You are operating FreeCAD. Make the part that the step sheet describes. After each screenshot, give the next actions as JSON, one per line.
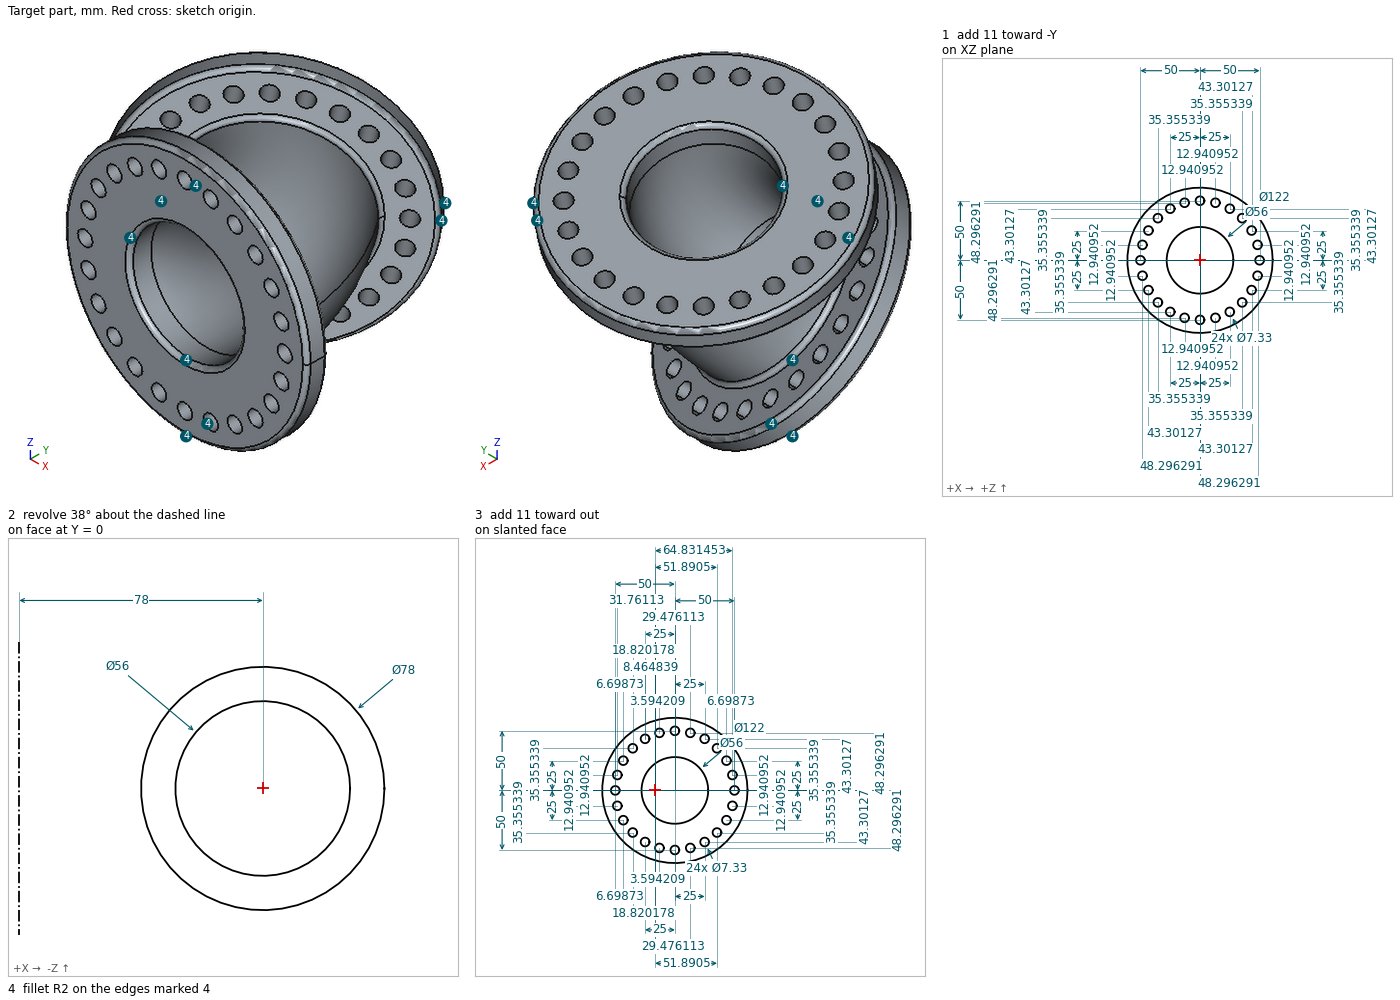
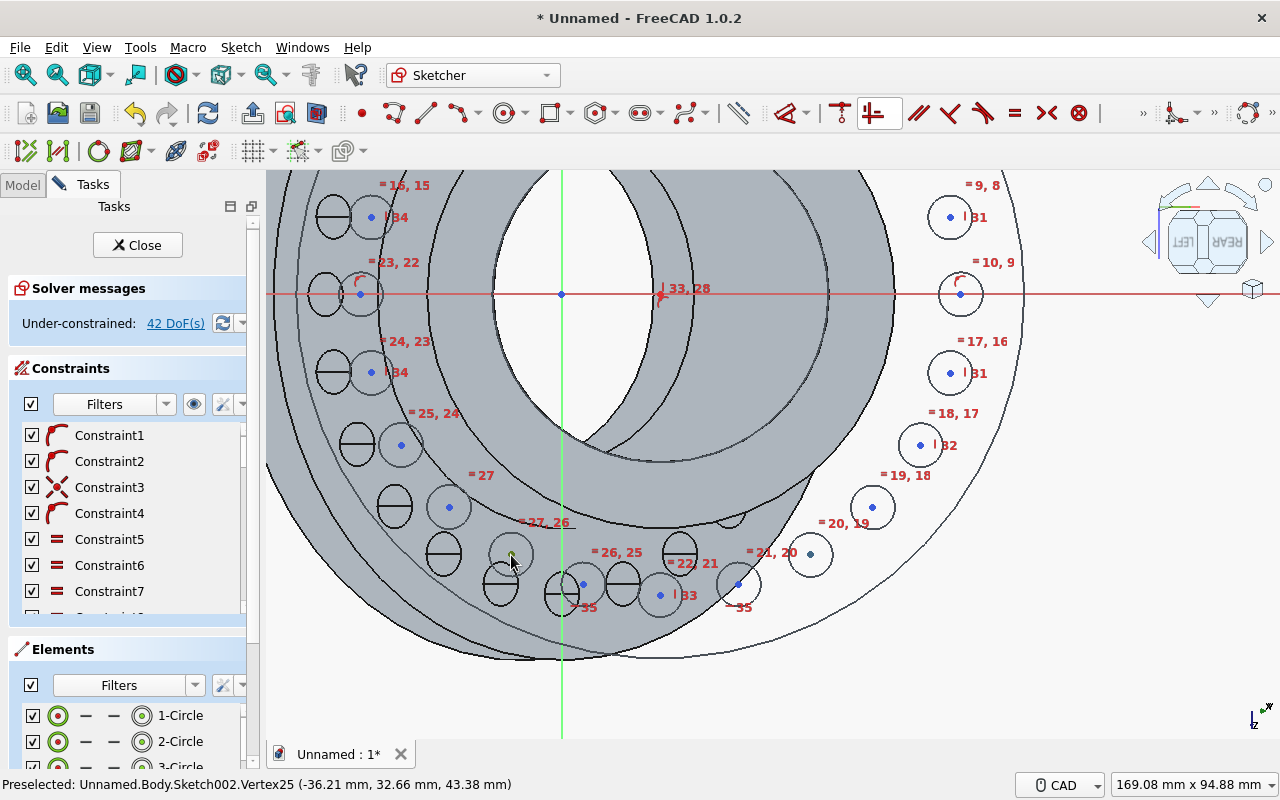
{"action": "left_click", "coordinate": [896, 114]}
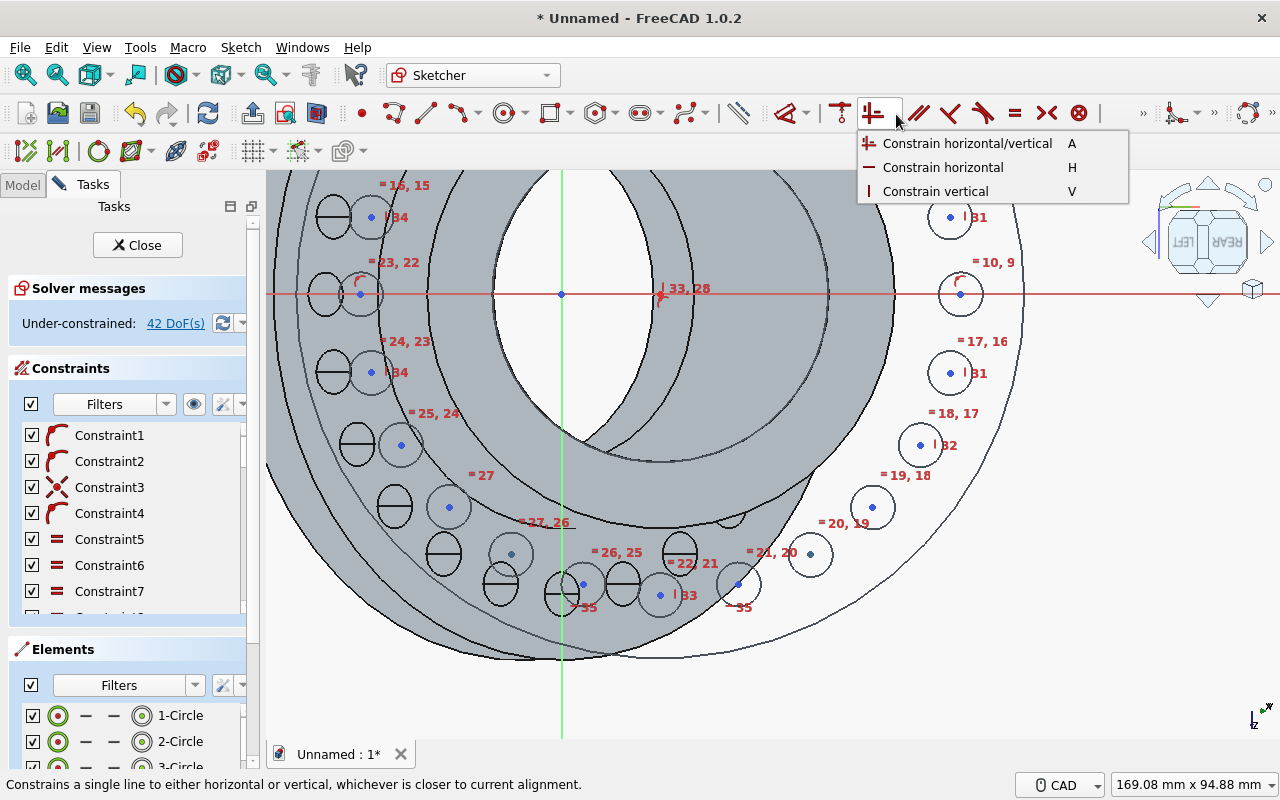
{"action": "left_click", "coordinate": [993, 167]}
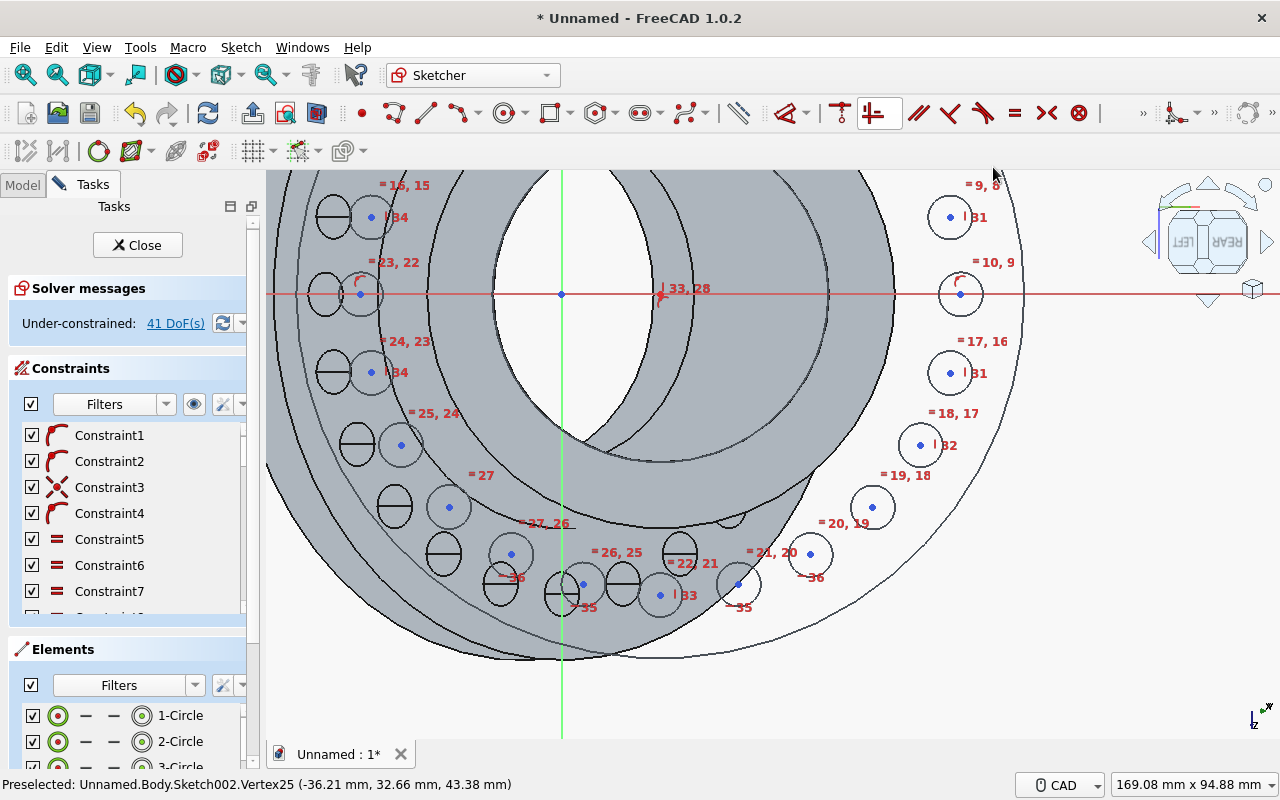
{"action": "left_click", "coordinate": [786, 114]}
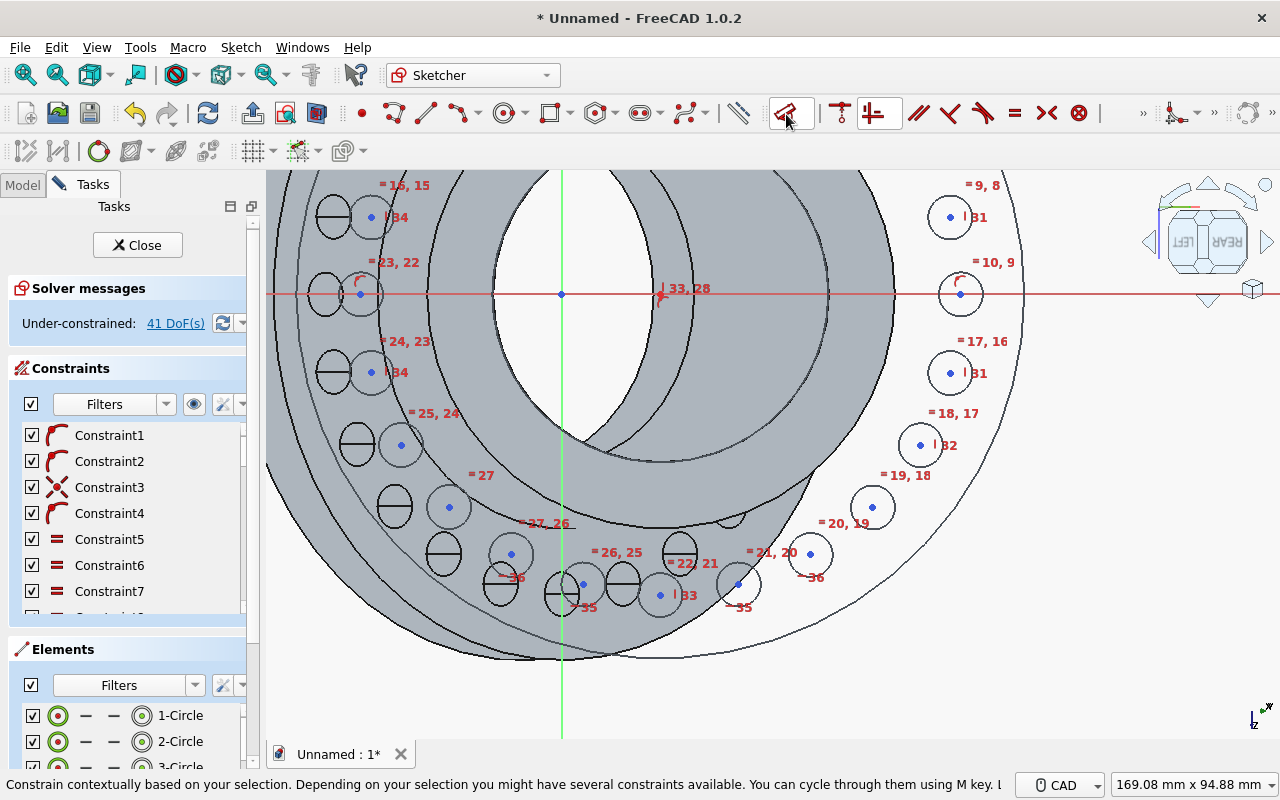
{"action": "left_click", "coordinate": [404, 553]}
{"action": "left_click", "coordinate": [381, 576]}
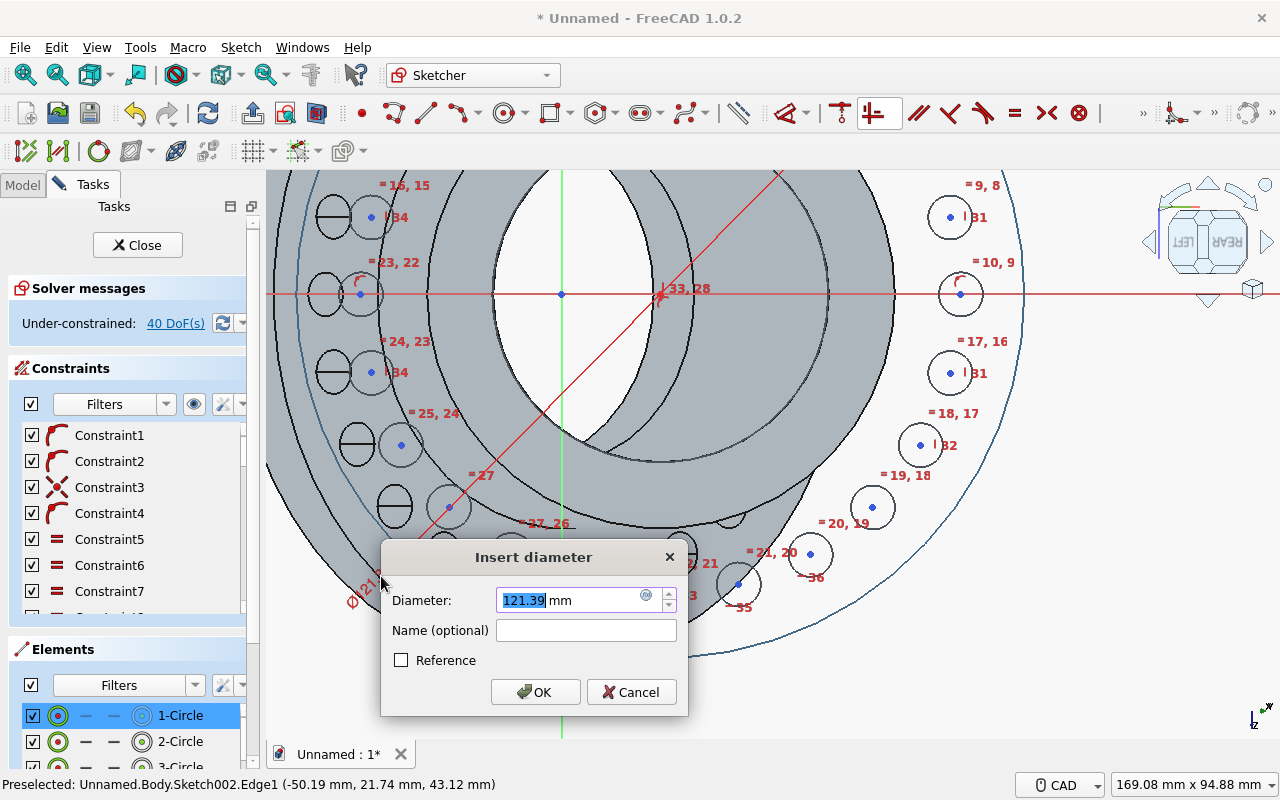
{"action": "type", "text": "122"}
{"action": "key", "text": "Return"}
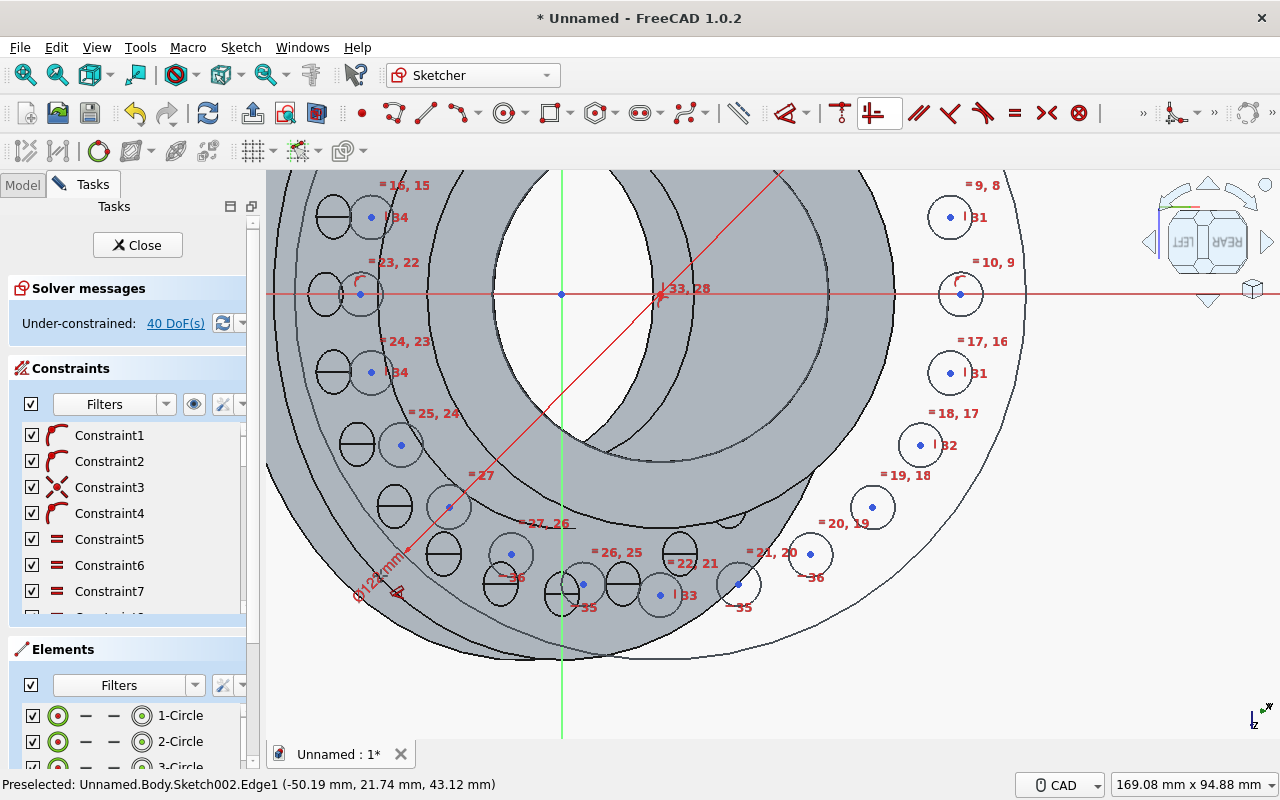
{"action": "scroll", "coordinate": [740, 585], "scroll_direction": "down", "scroll_amount": 4}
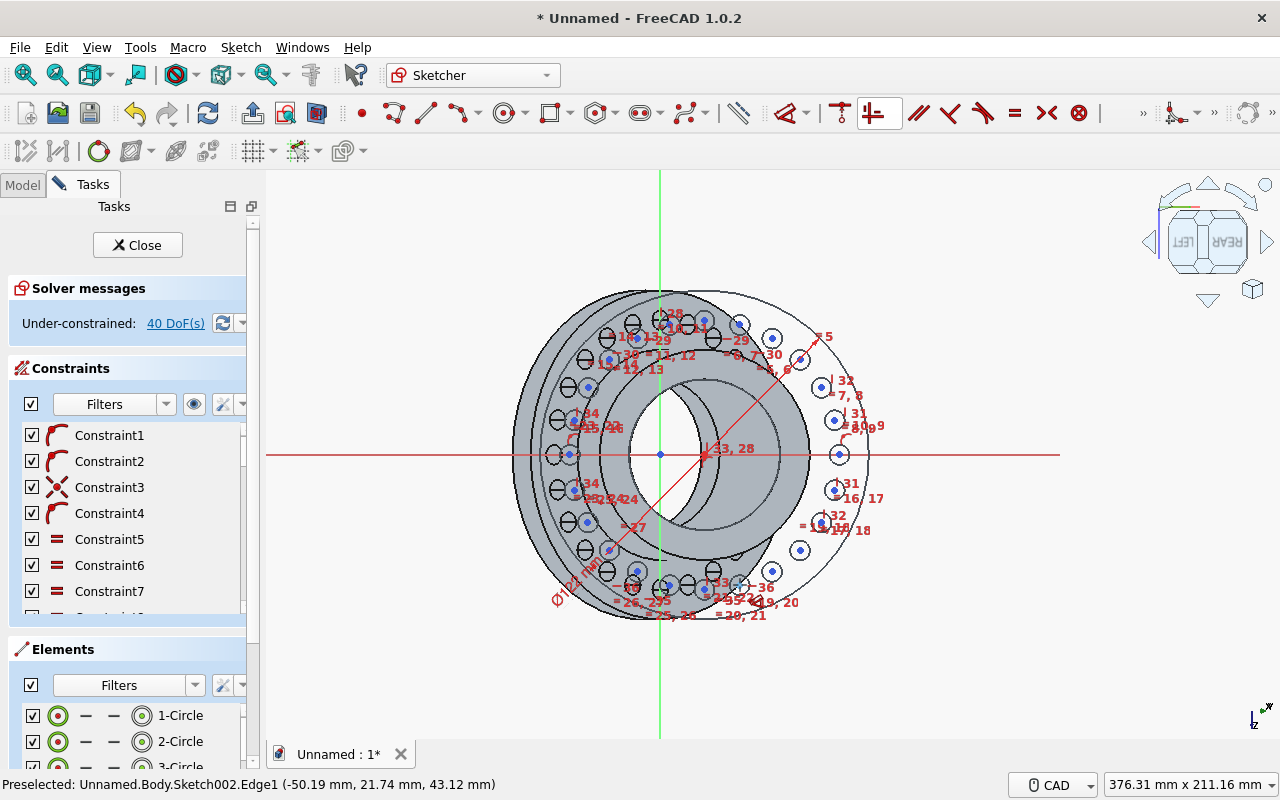
{"action": "scroll", "coordinate": [807, 353], "scroll_direction": "up", "scroll_amount": 4}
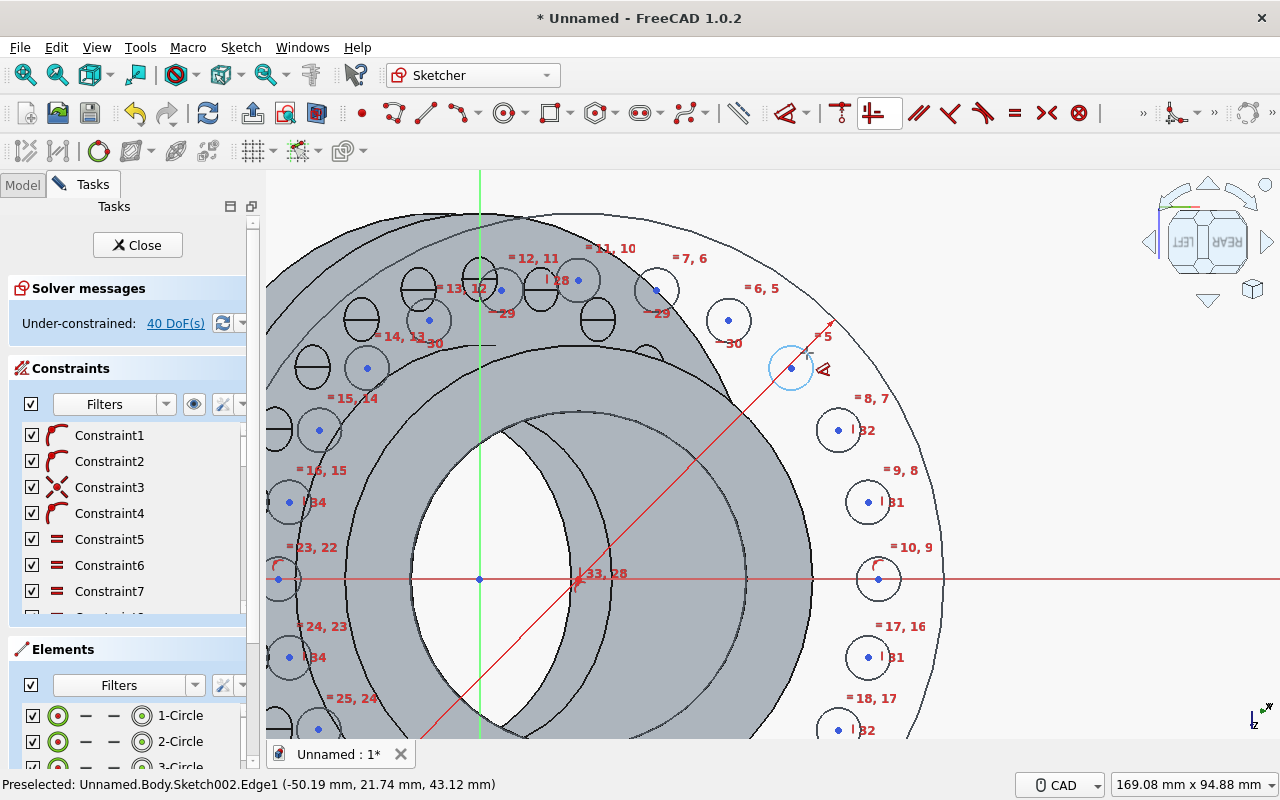
{"action": "left_click", "coordinate": [807, 352]}
{"action": "left_click", "coordinate": [843, 352]}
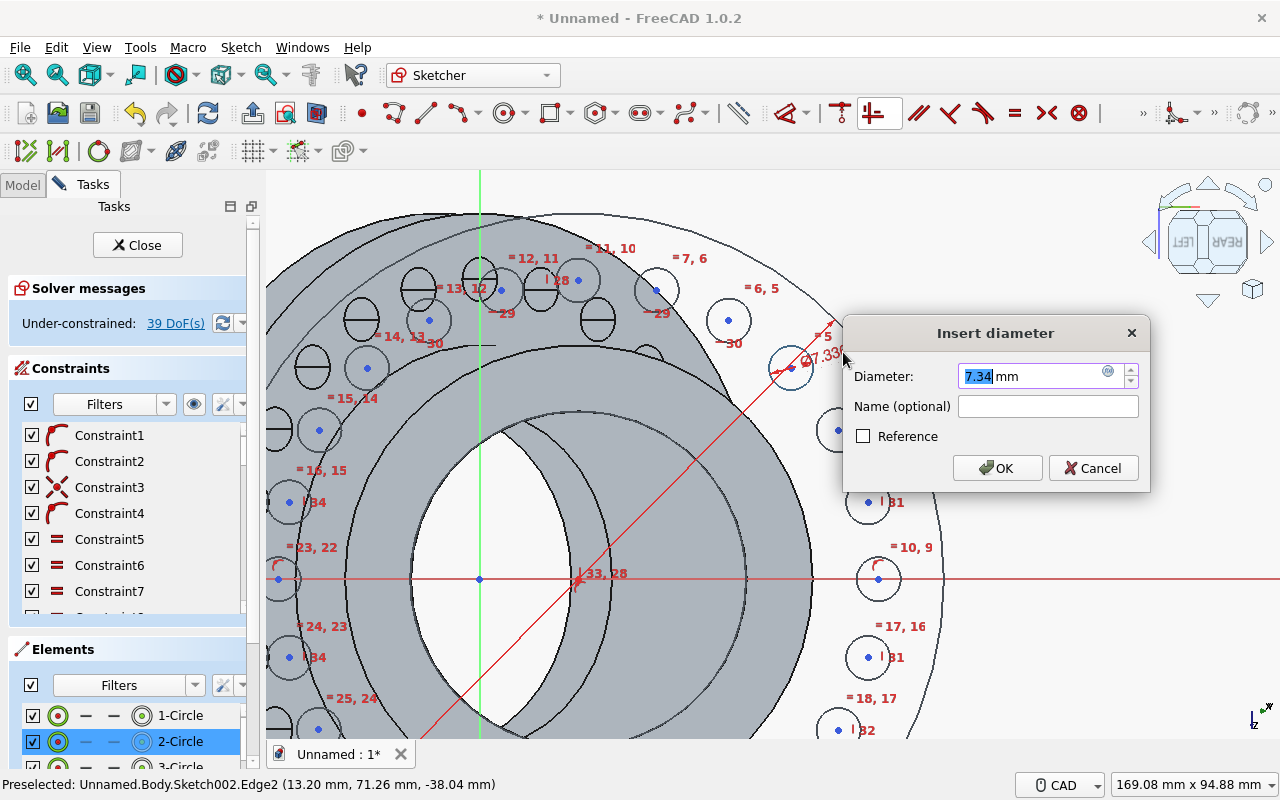
{"action": "type", "text": "7.33"}
{"action": "key", "text": "Return"}